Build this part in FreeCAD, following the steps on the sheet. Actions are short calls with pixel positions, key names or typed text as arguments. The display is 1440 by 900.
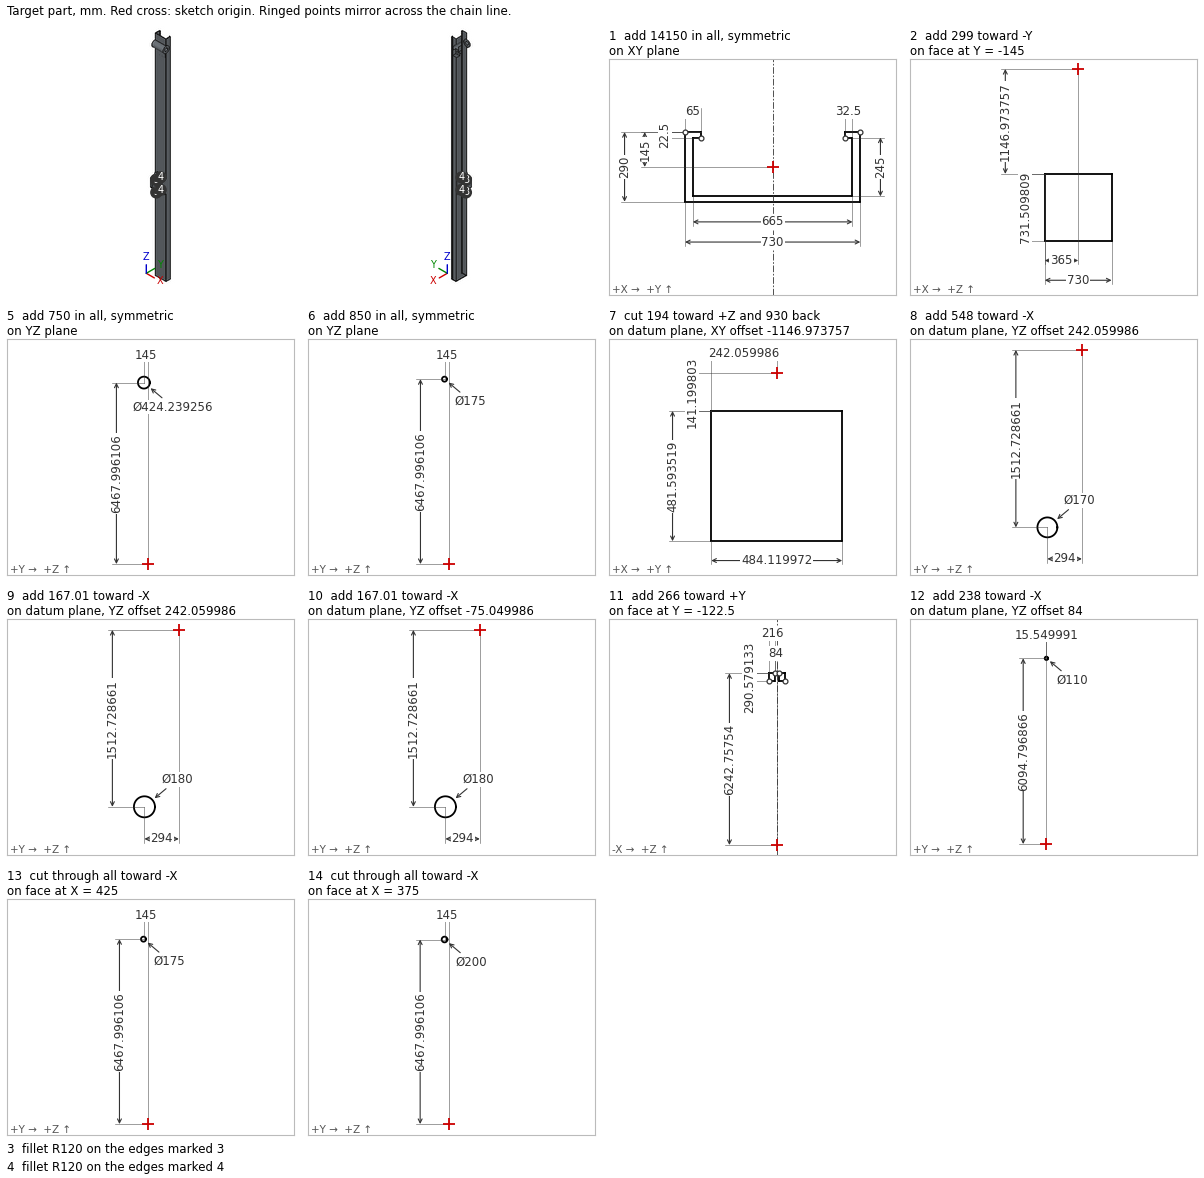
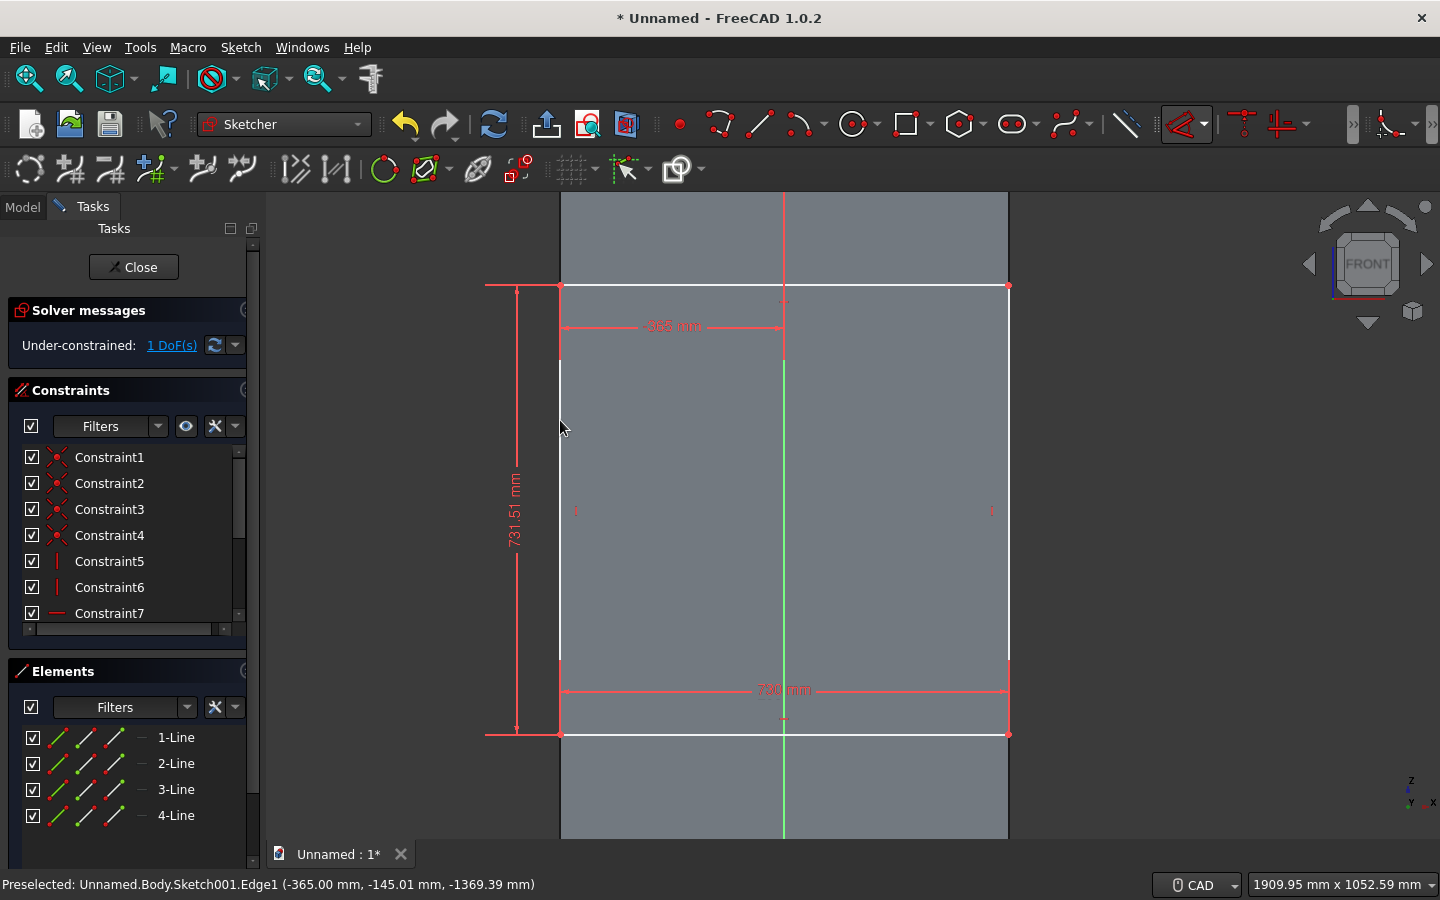
click(560, 285)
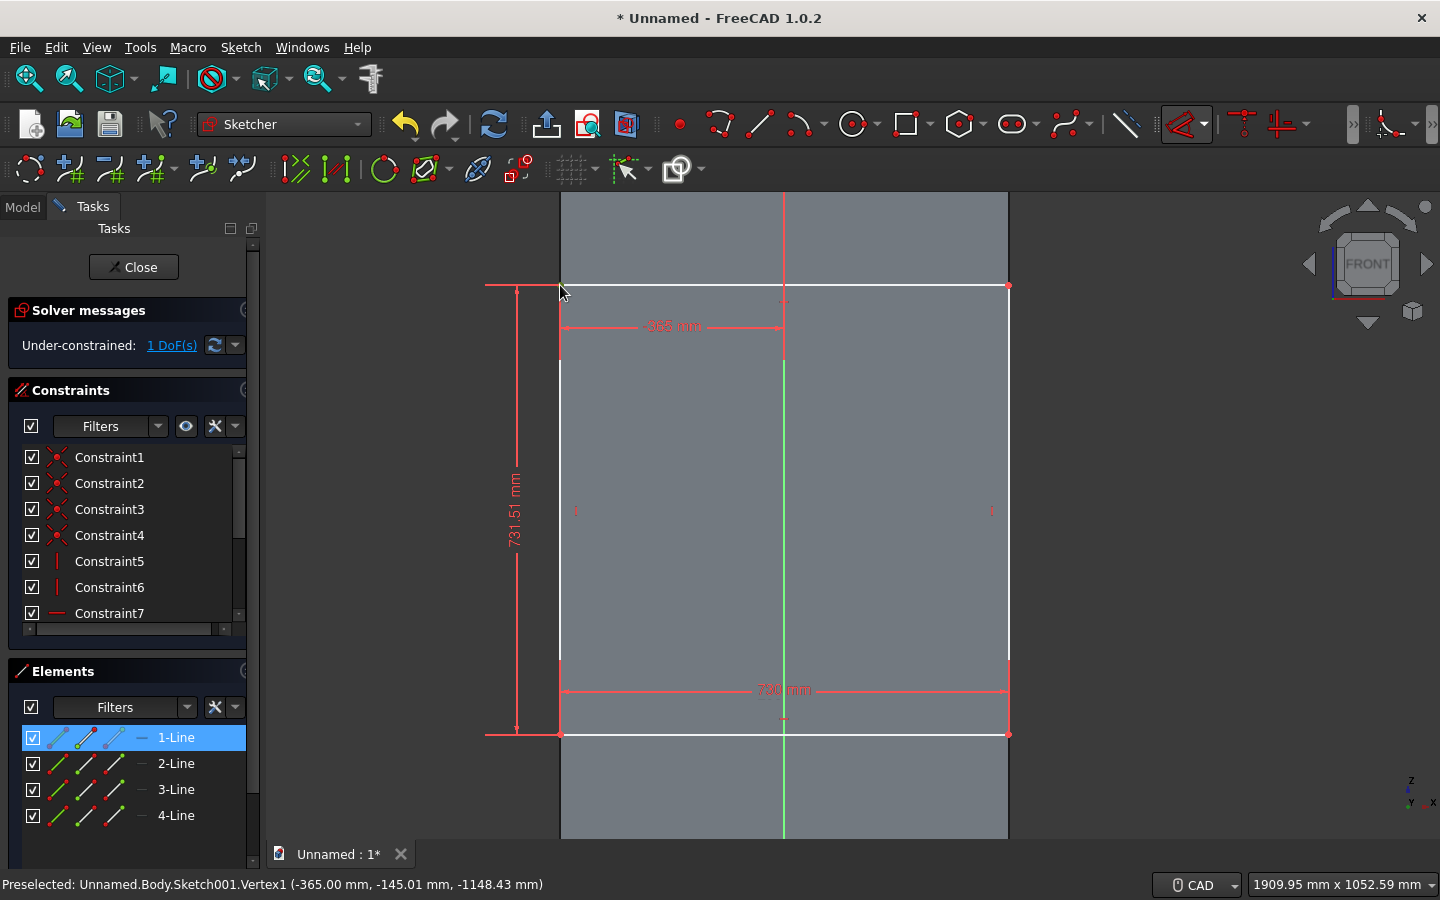
key(i)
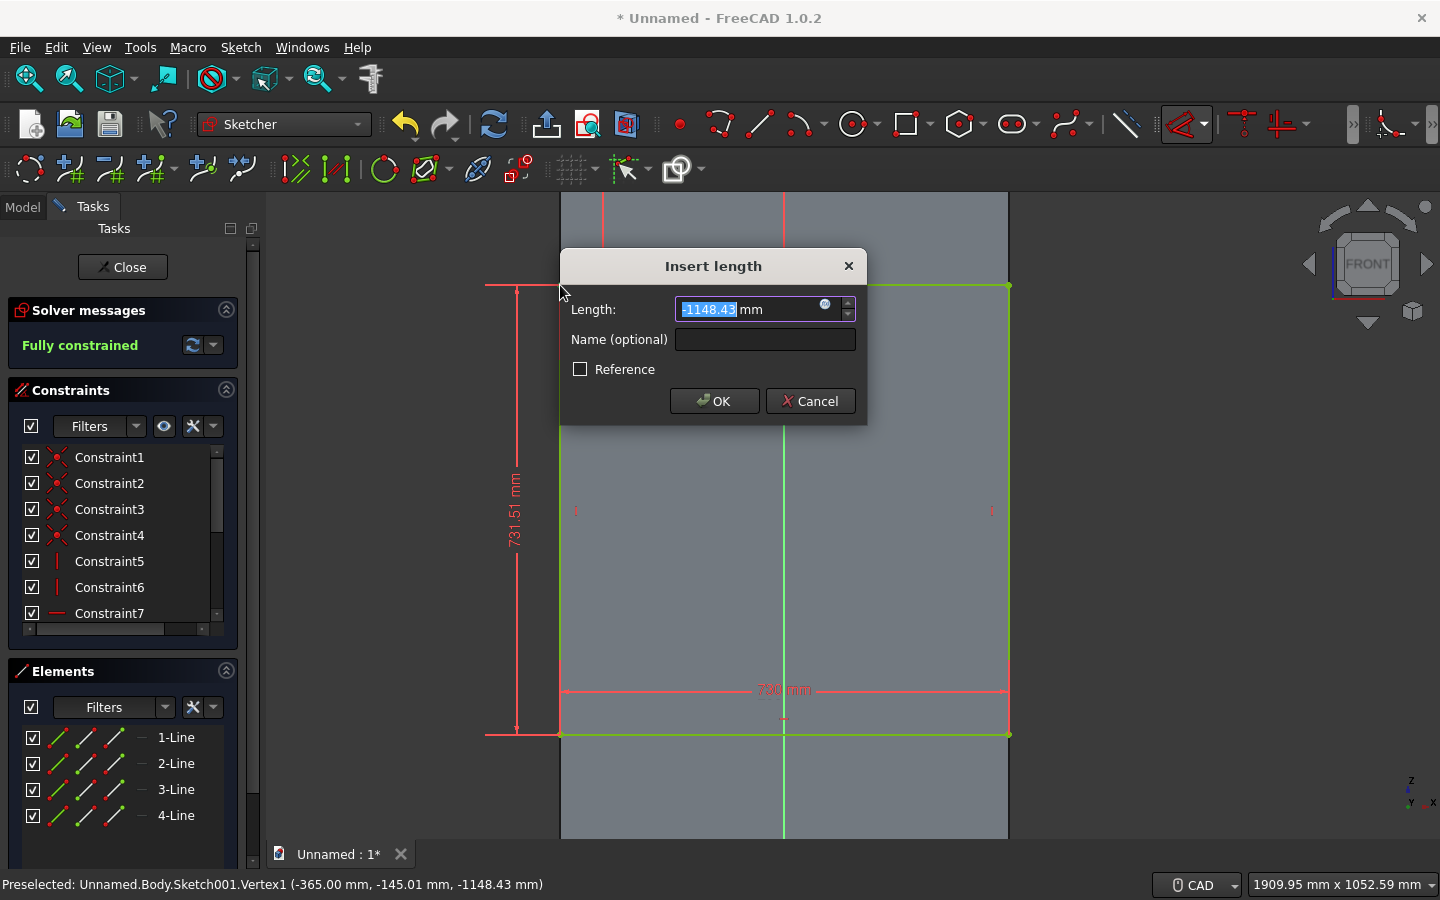
text(-1146.973757)
key(Return)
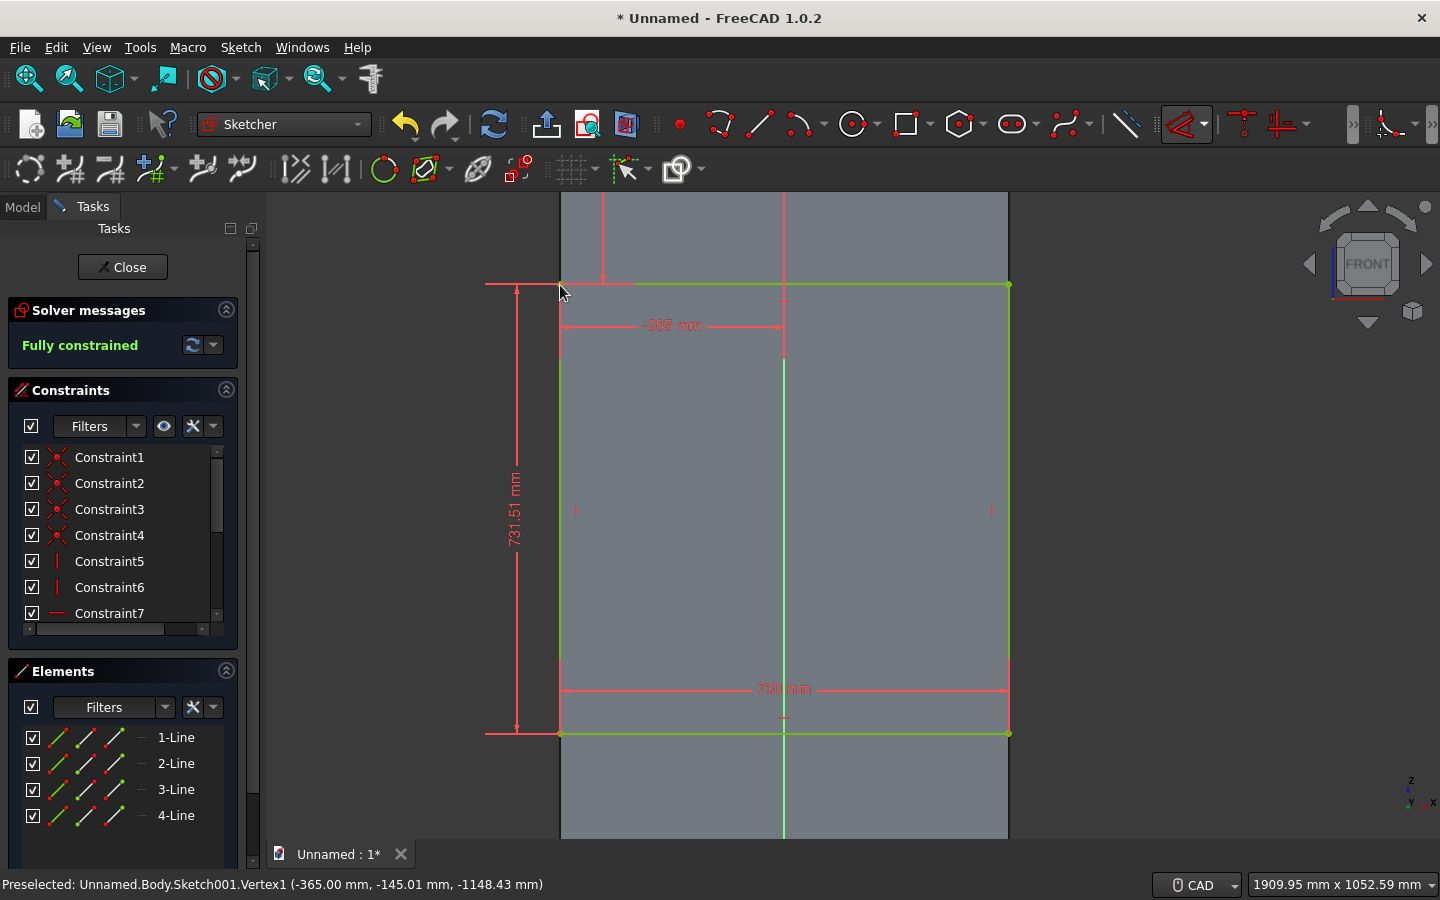
click(123, 267)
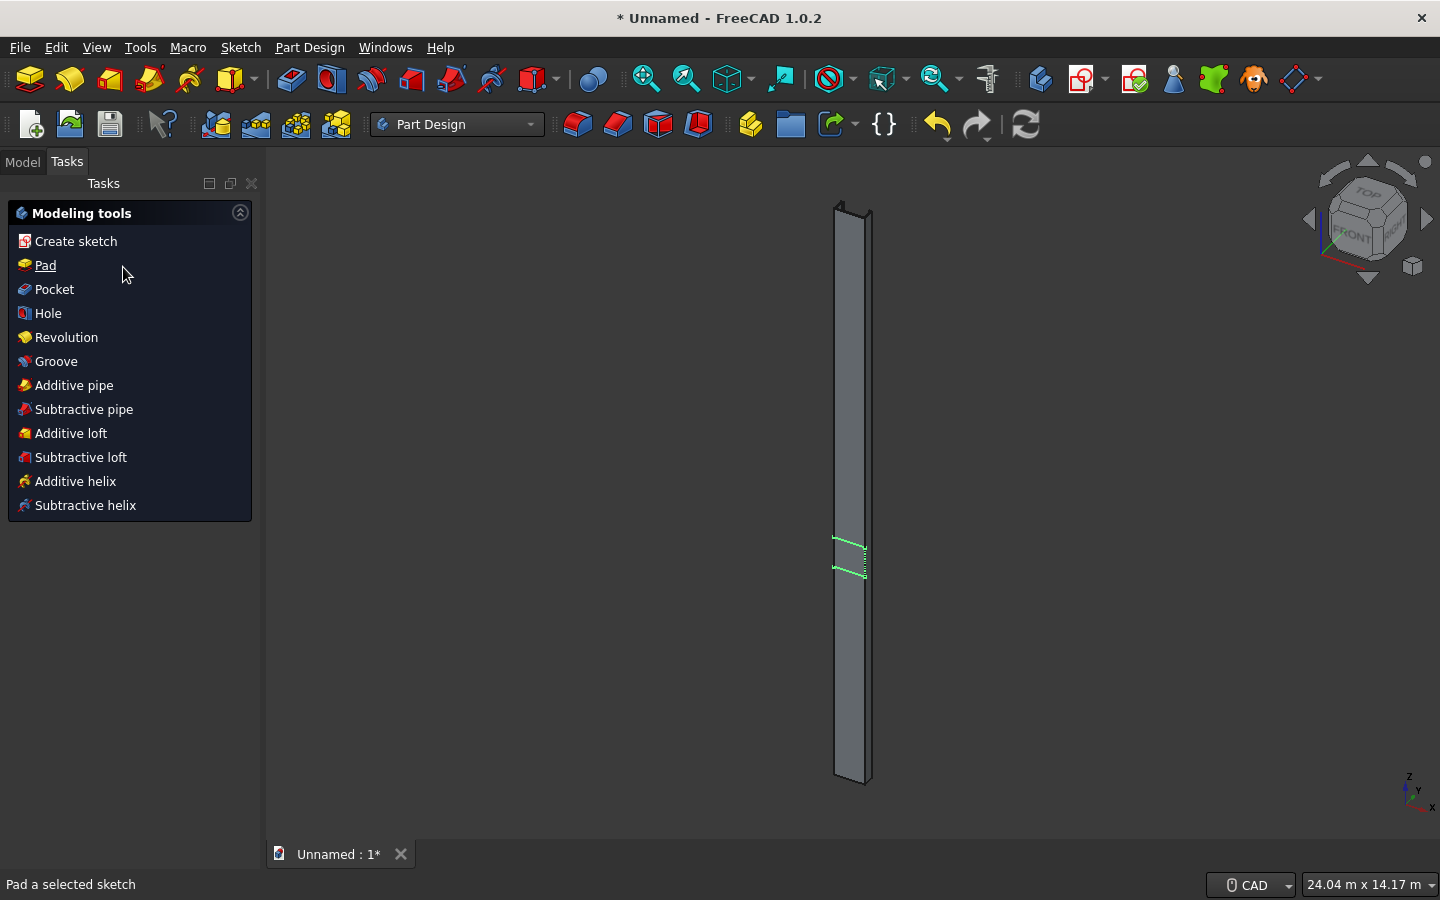
click(30, 80)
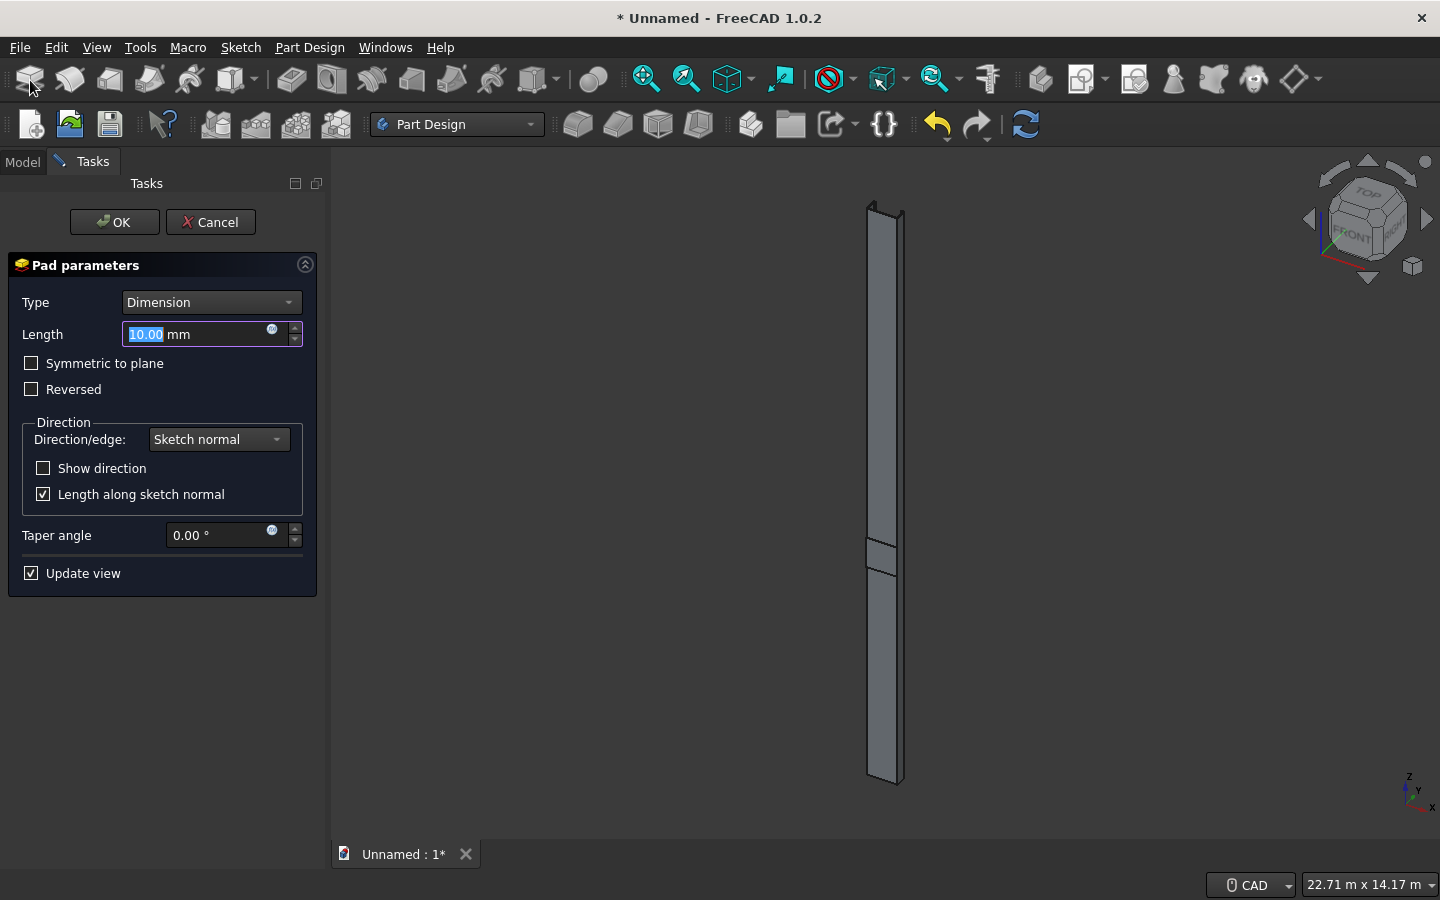
text(299)
key(Tab)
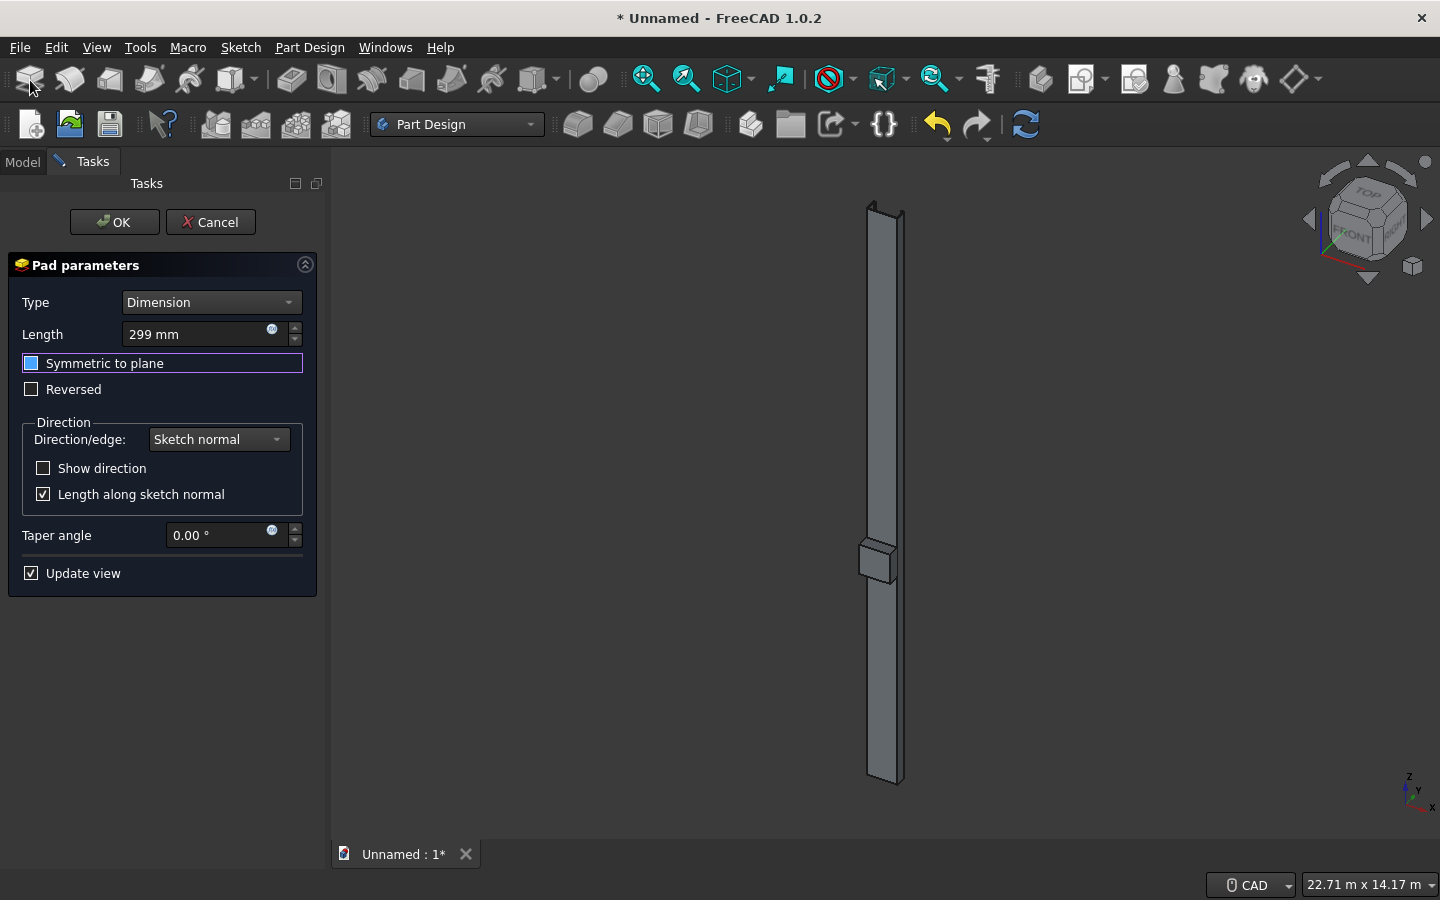
click(115, 222)